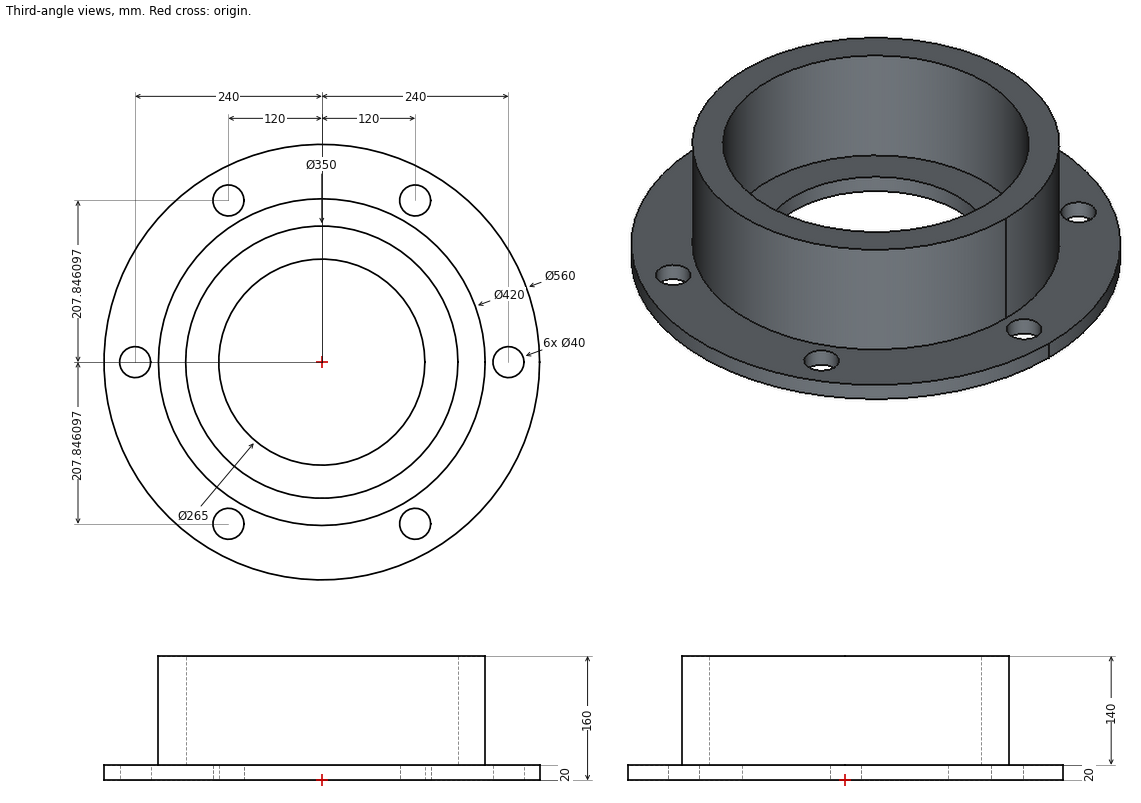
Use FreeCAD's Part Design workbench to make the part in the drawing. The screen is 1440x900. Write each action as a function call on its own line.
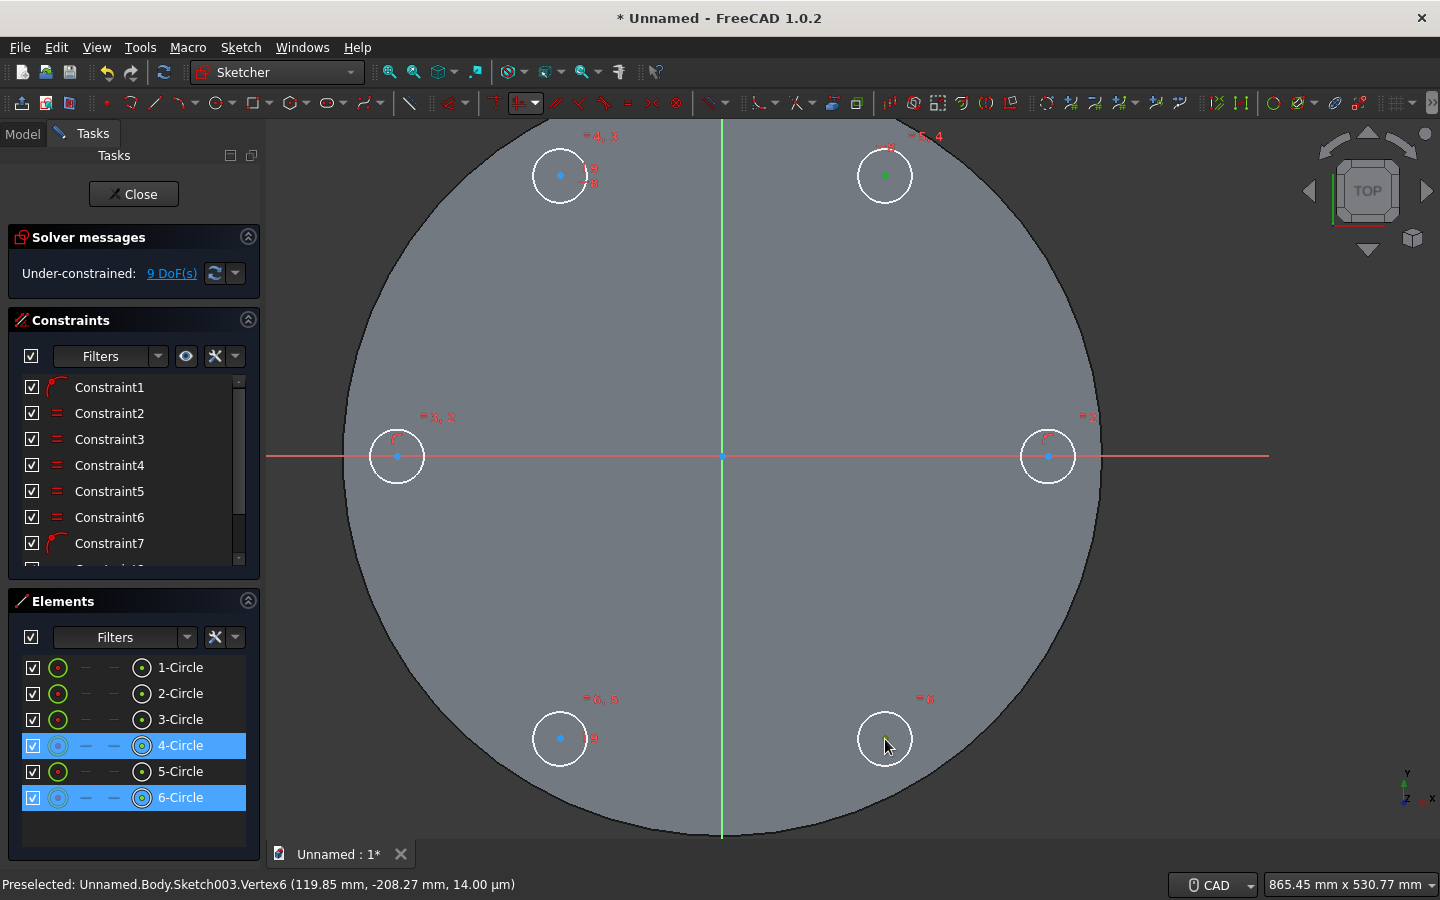
key(v)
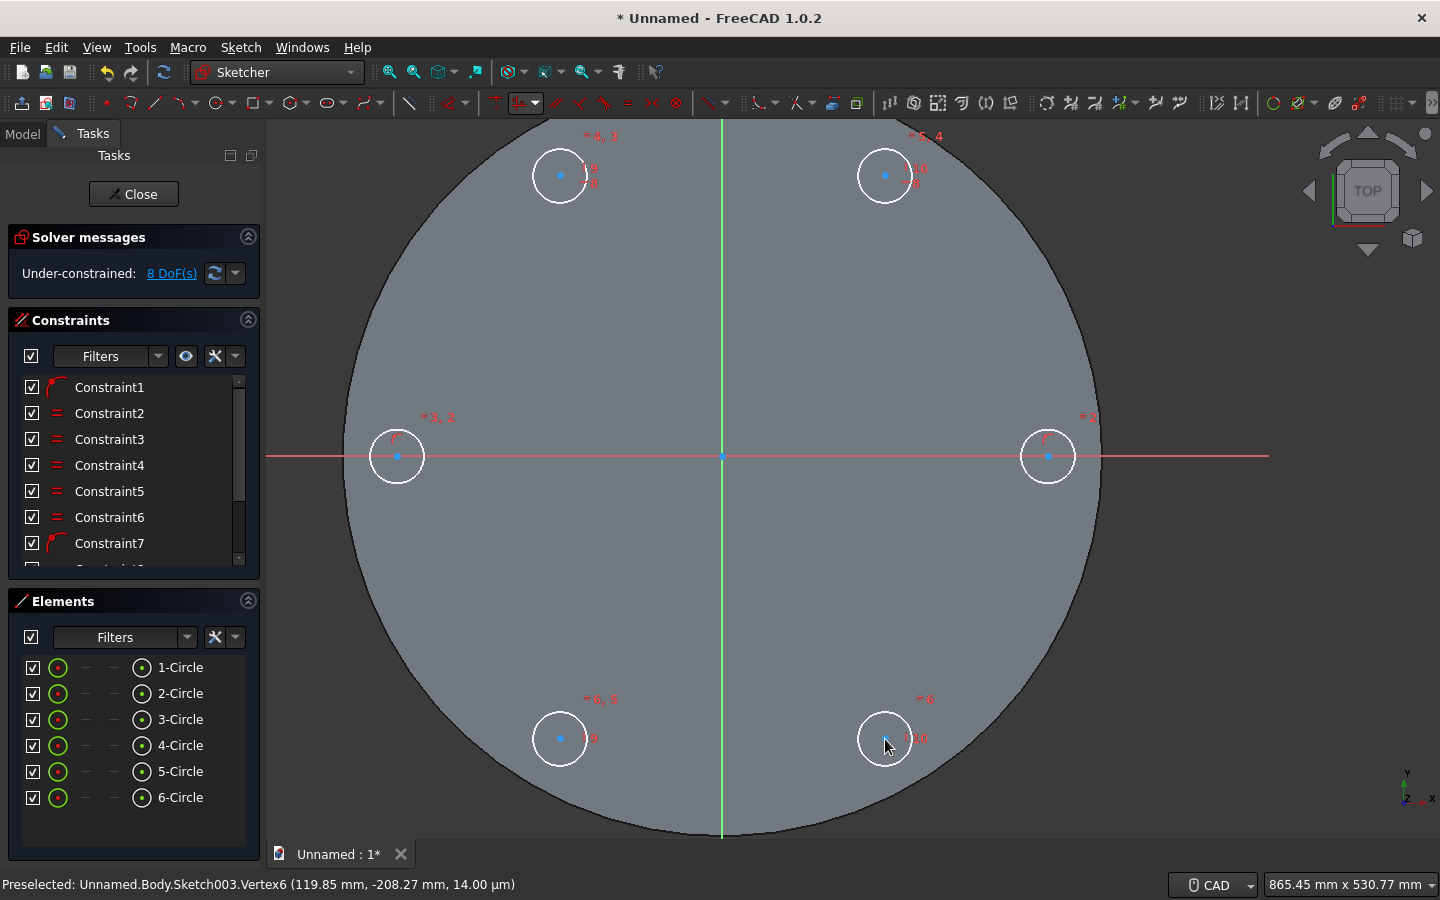
click(560, 739)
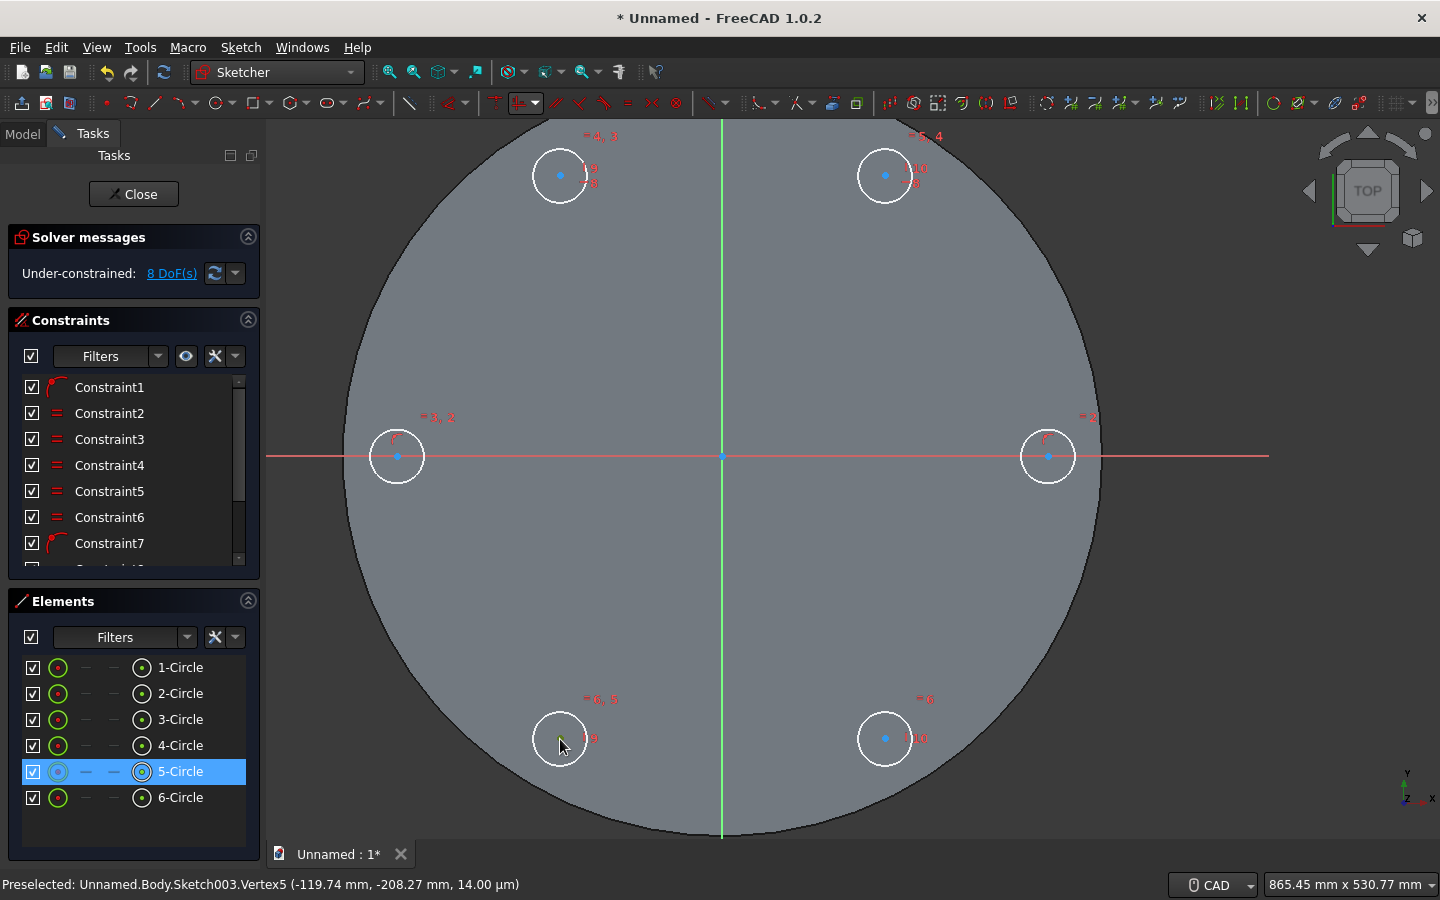
click(885, 739)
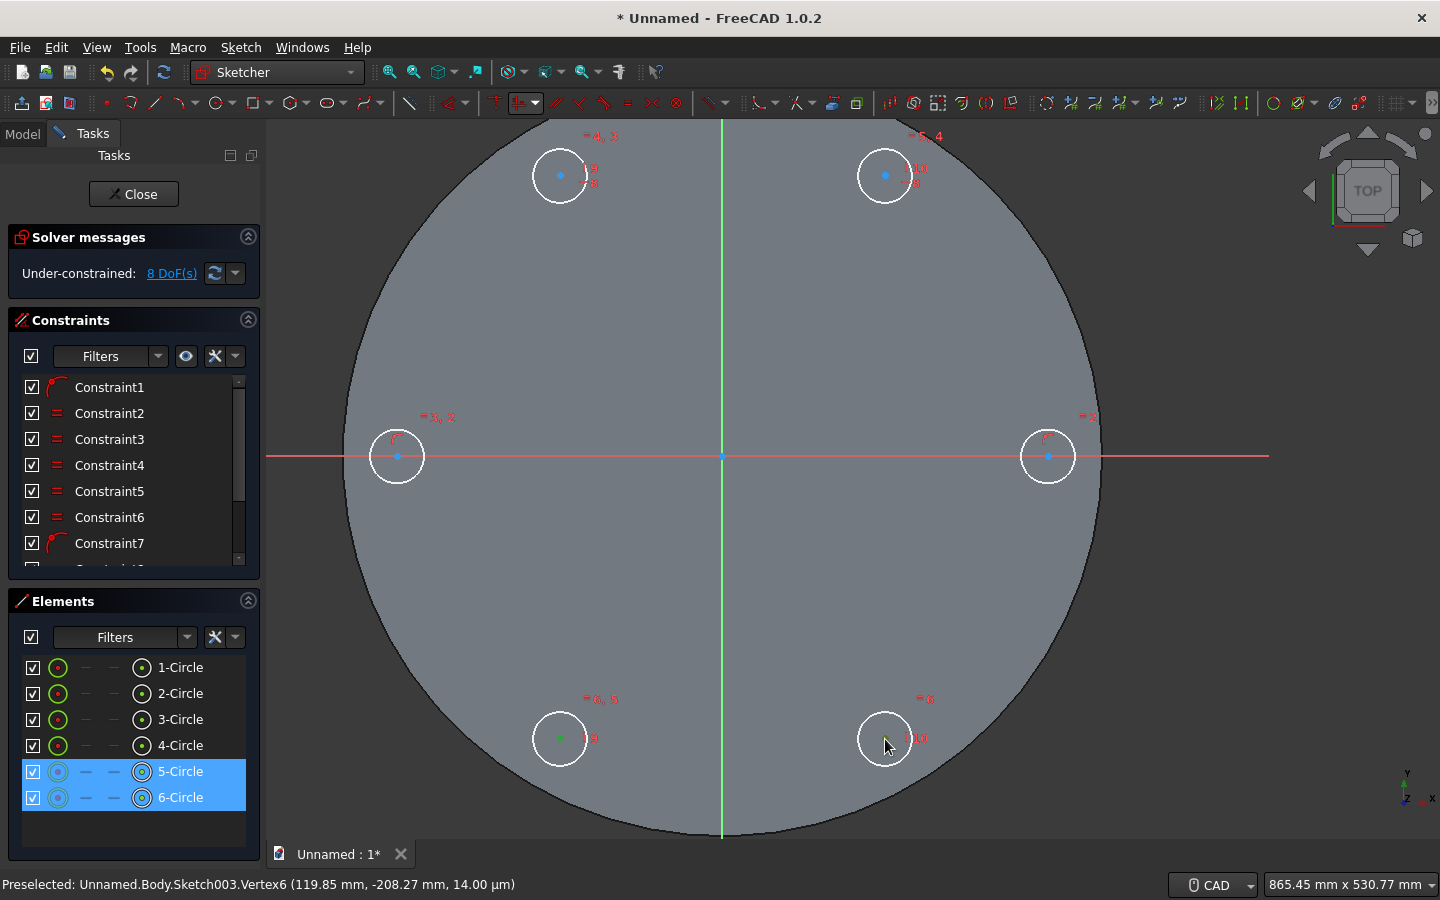
key(h)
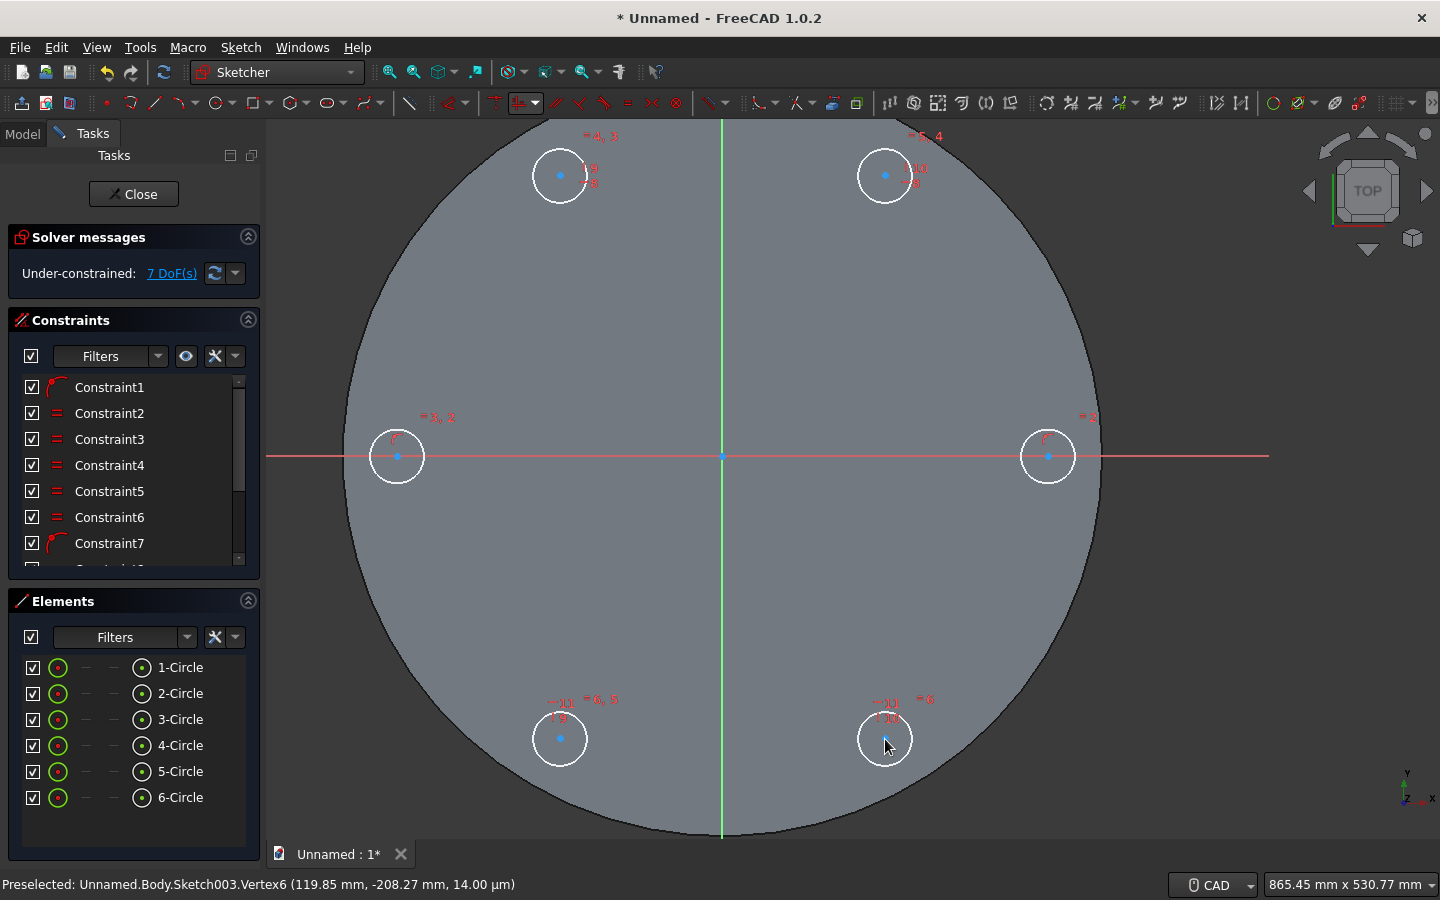
click(448, 104)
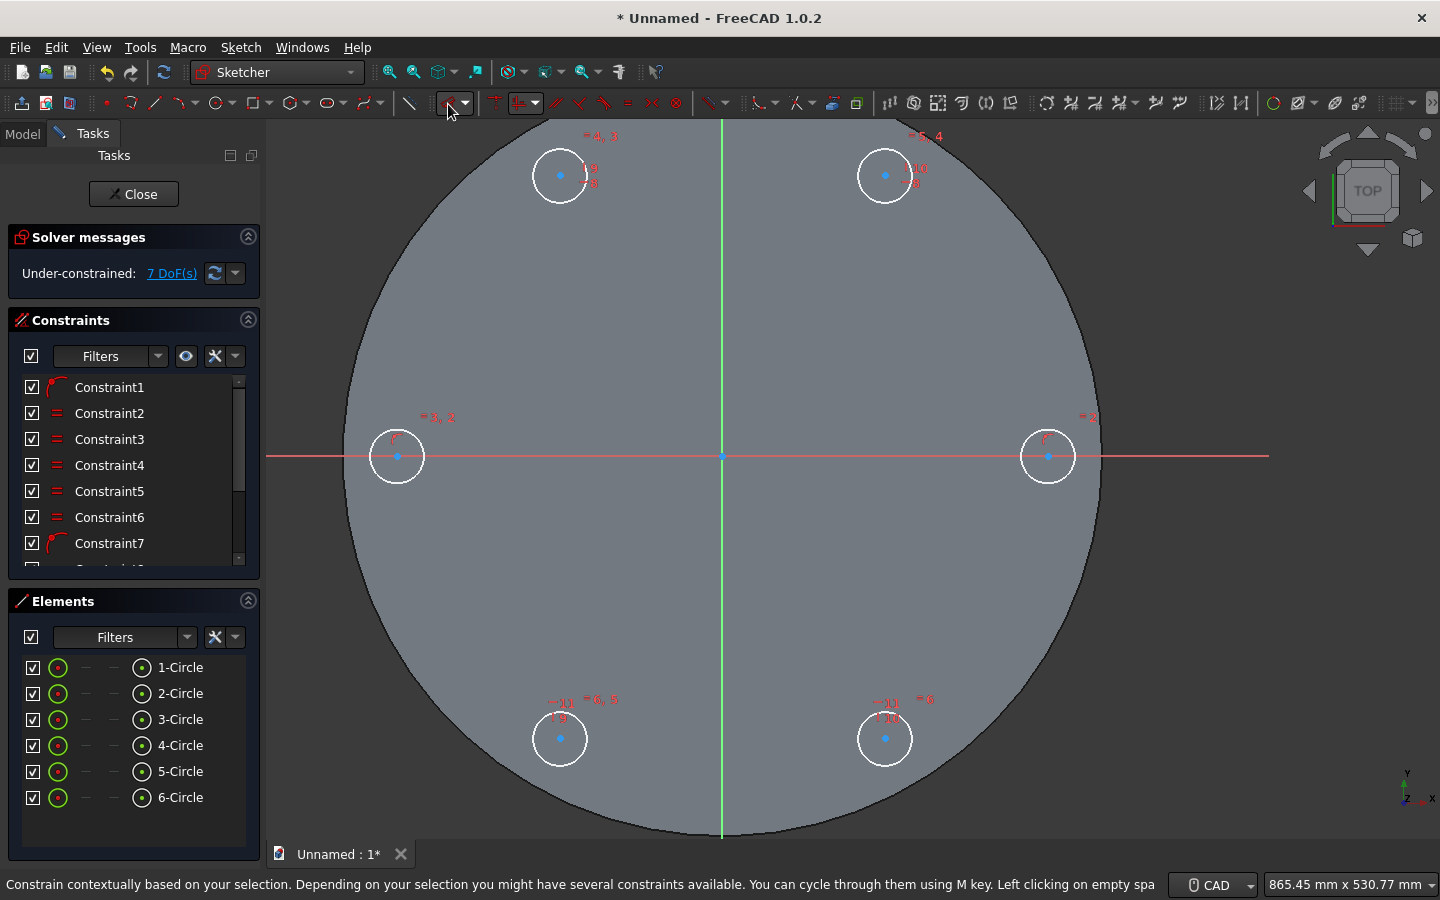
click(1067, 437)
click(1089, 414)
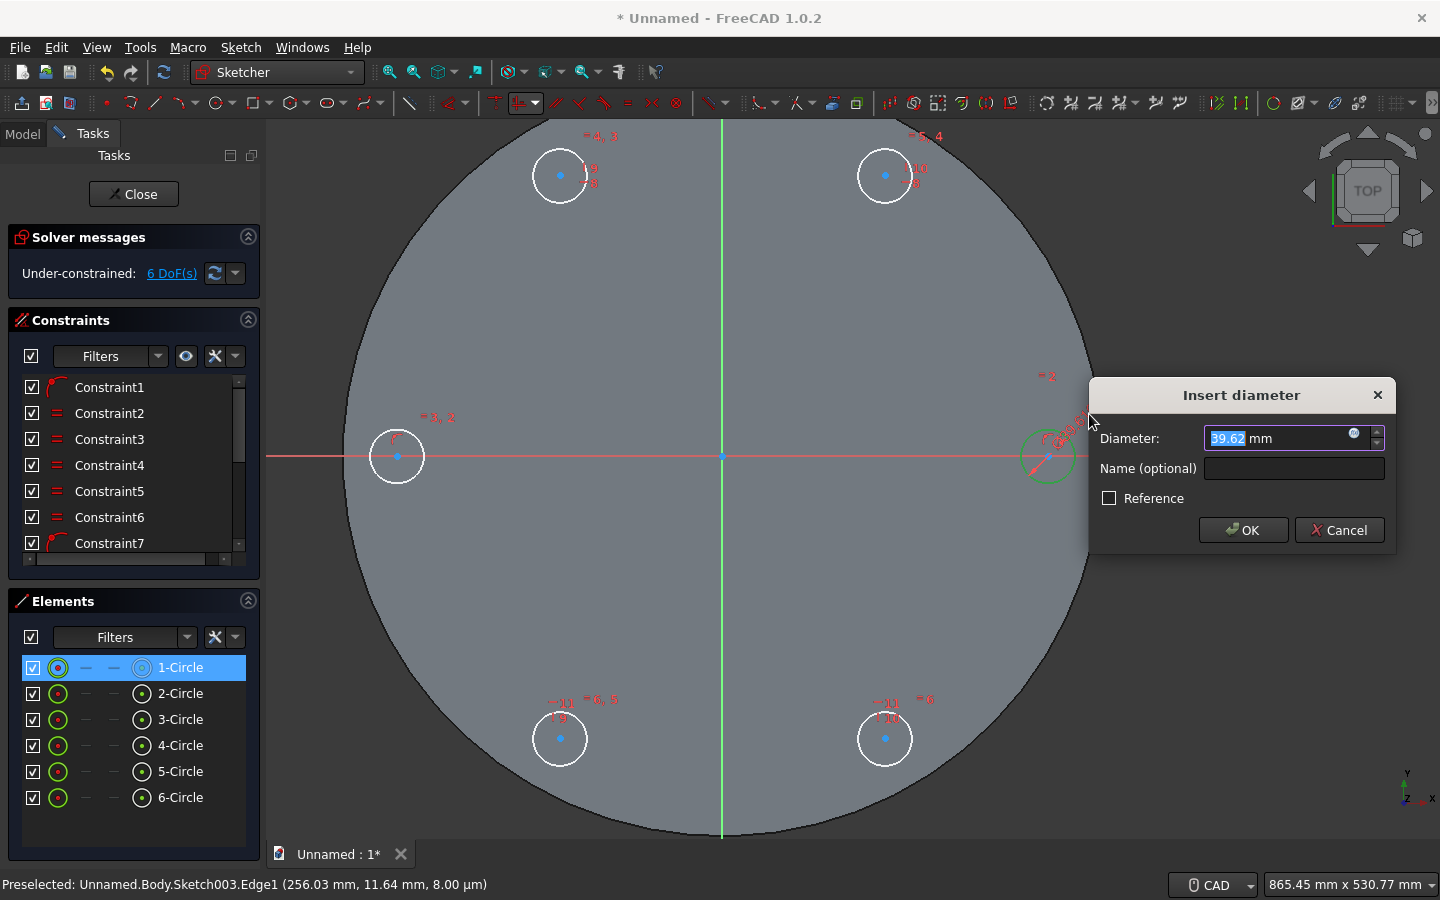
text(40)
key(Return)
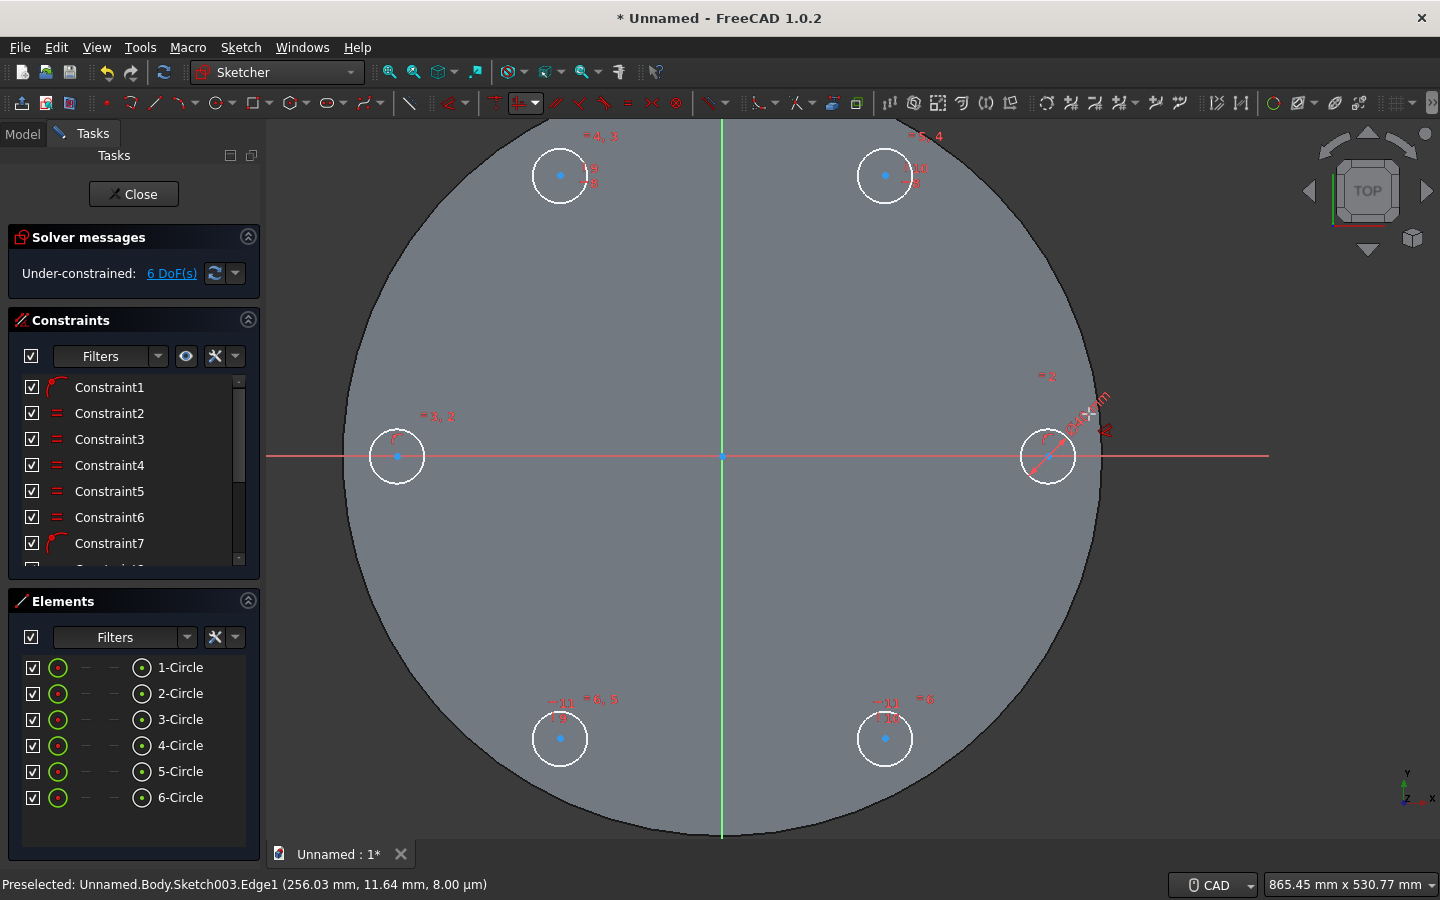
click(1048, 456)
click(885, 490)